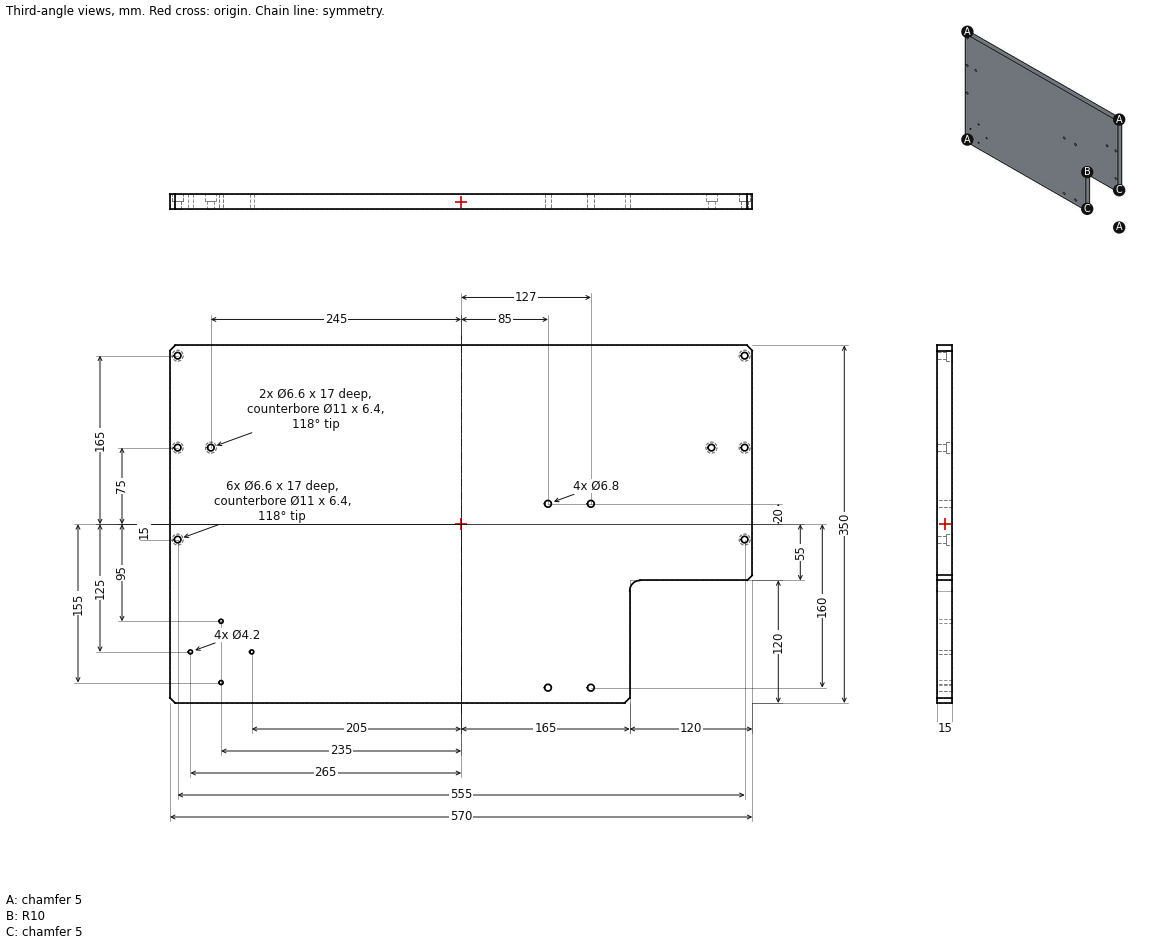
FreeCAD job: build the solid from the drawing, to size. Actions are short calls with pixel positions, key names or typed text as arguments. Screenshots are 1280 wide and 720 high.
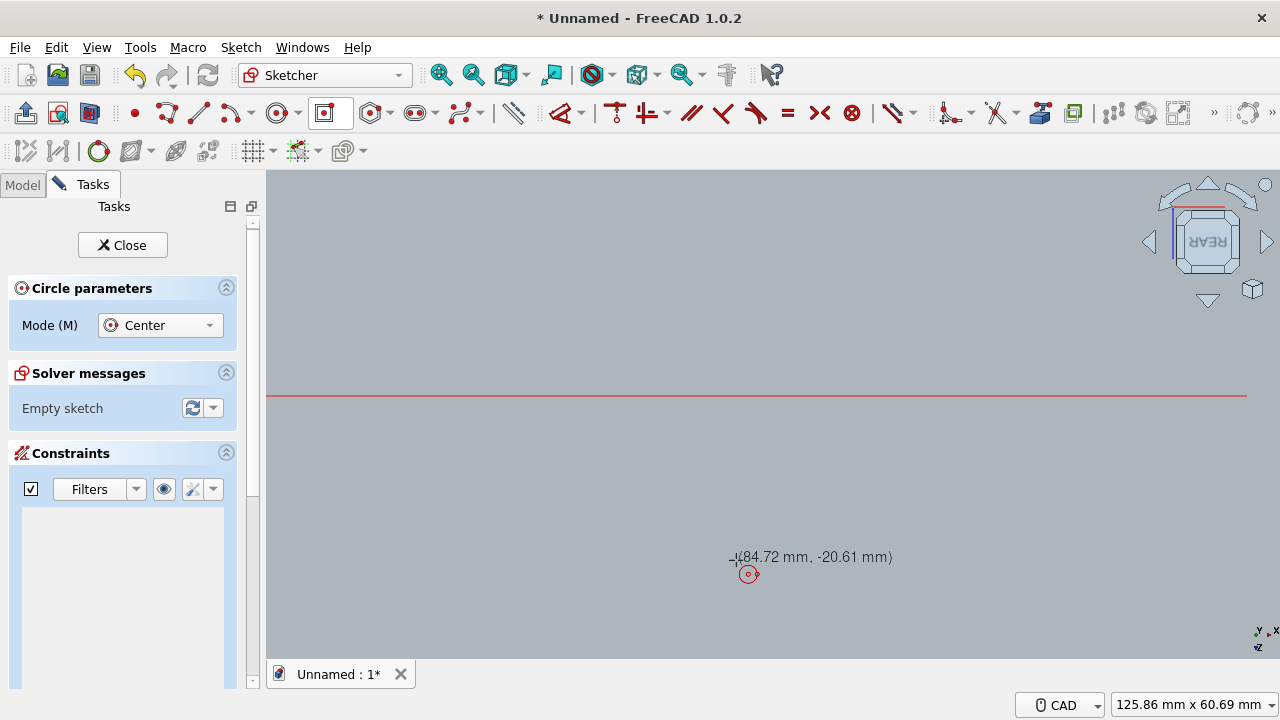
scroll(737, 562, down, 8)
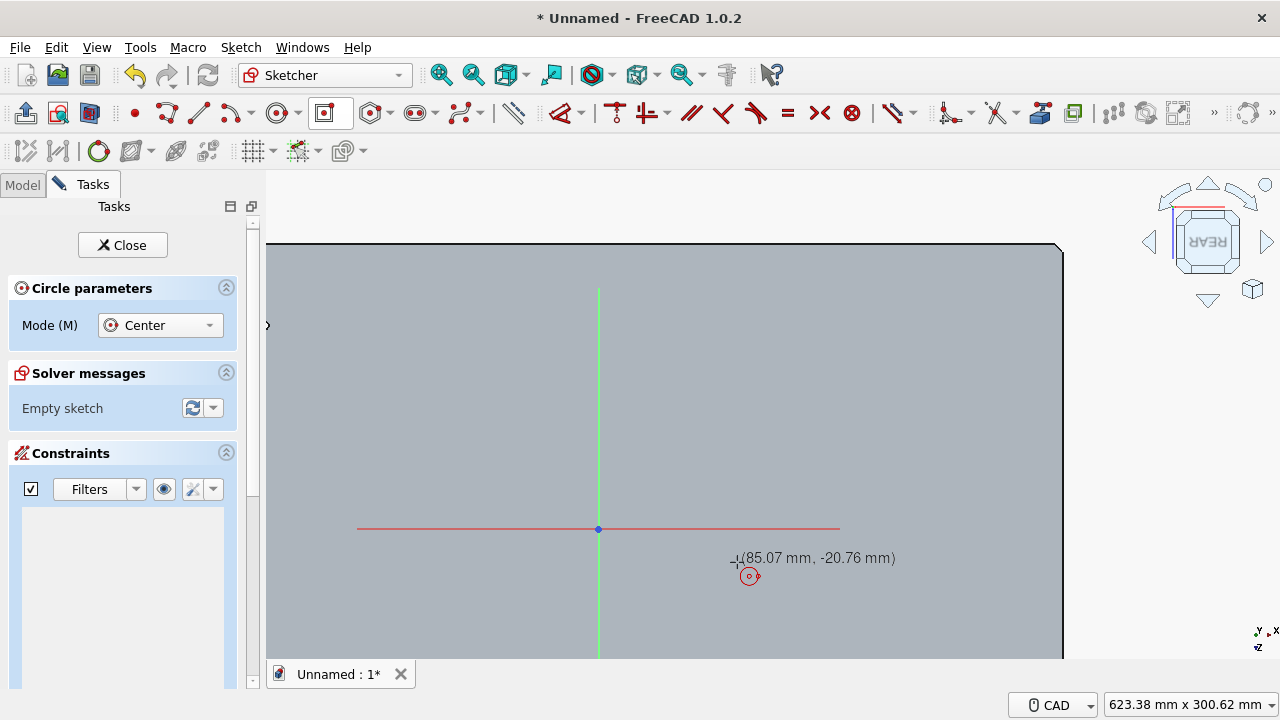
click(737, 562)
move(741, 558)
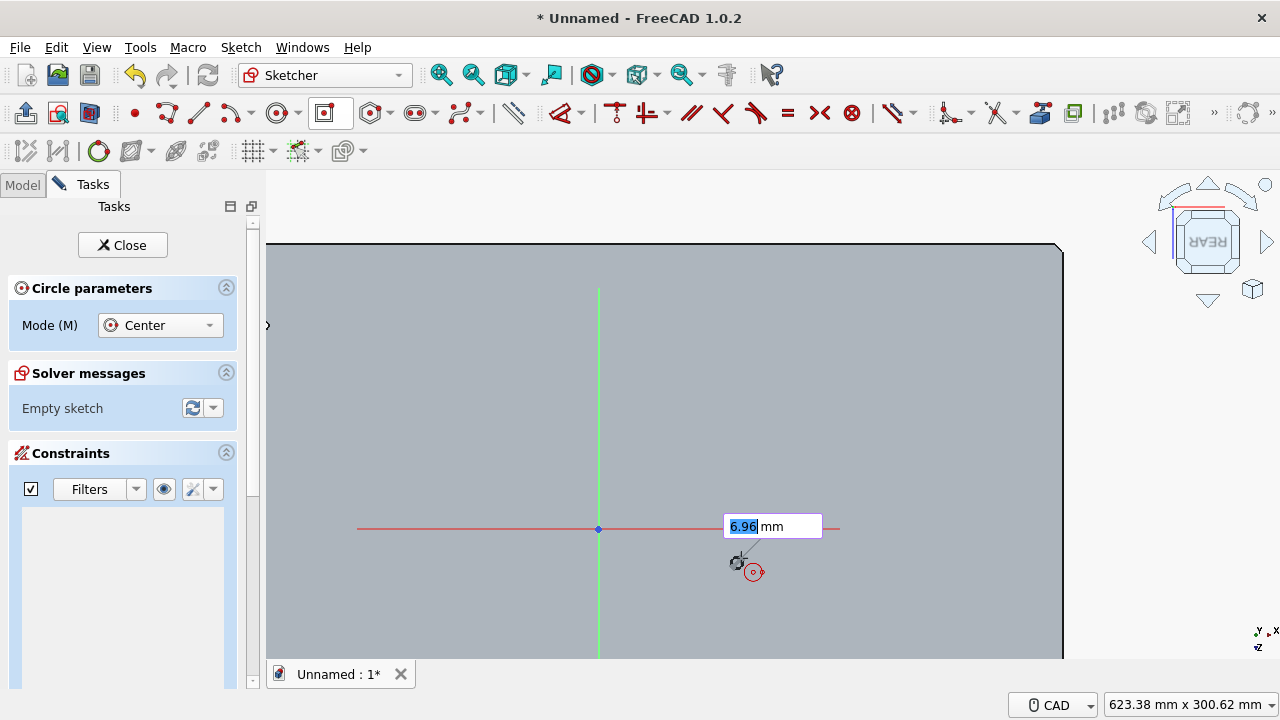
text(6.8)
key(Return)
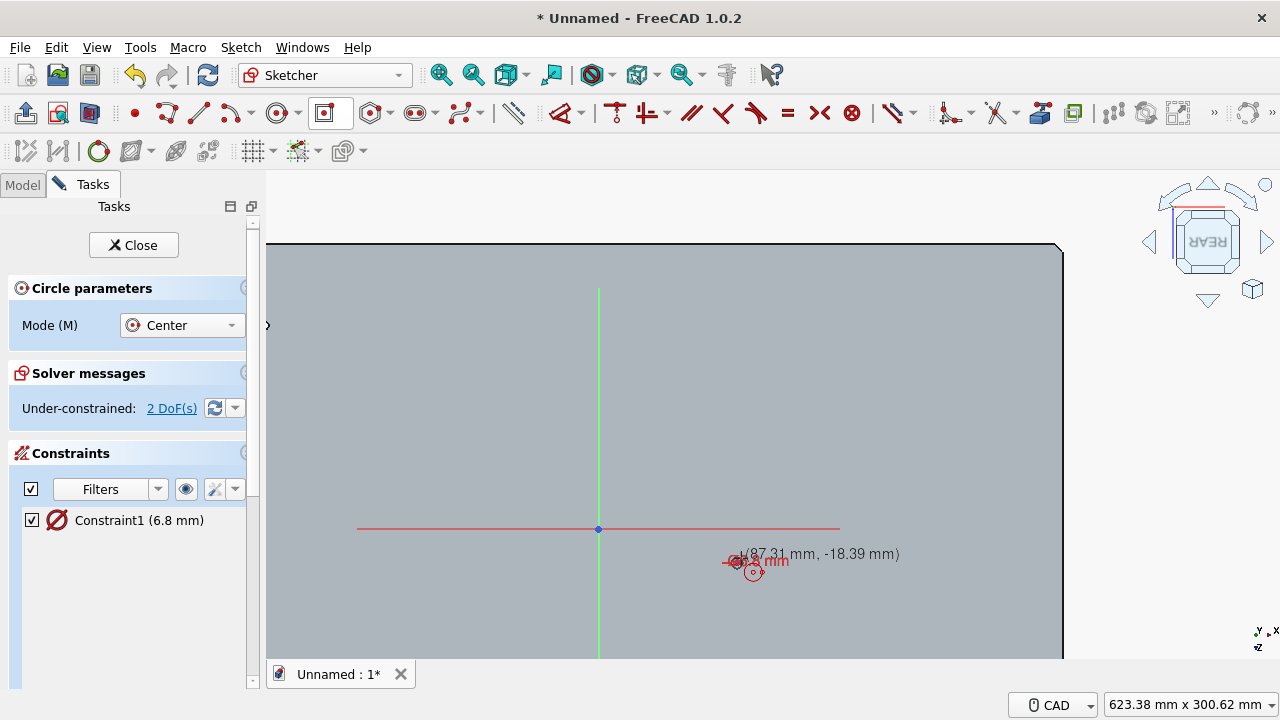
scroll(806, 562, up, 8)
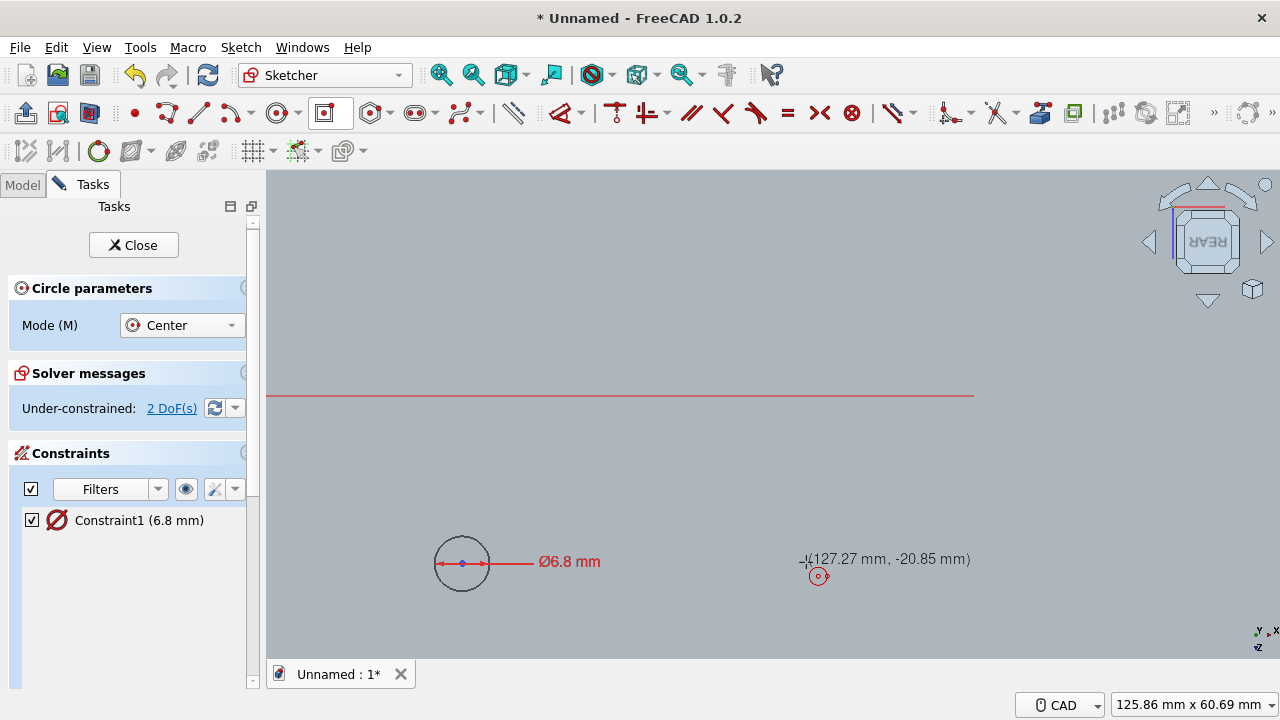
scroll(806, 562, down, 8)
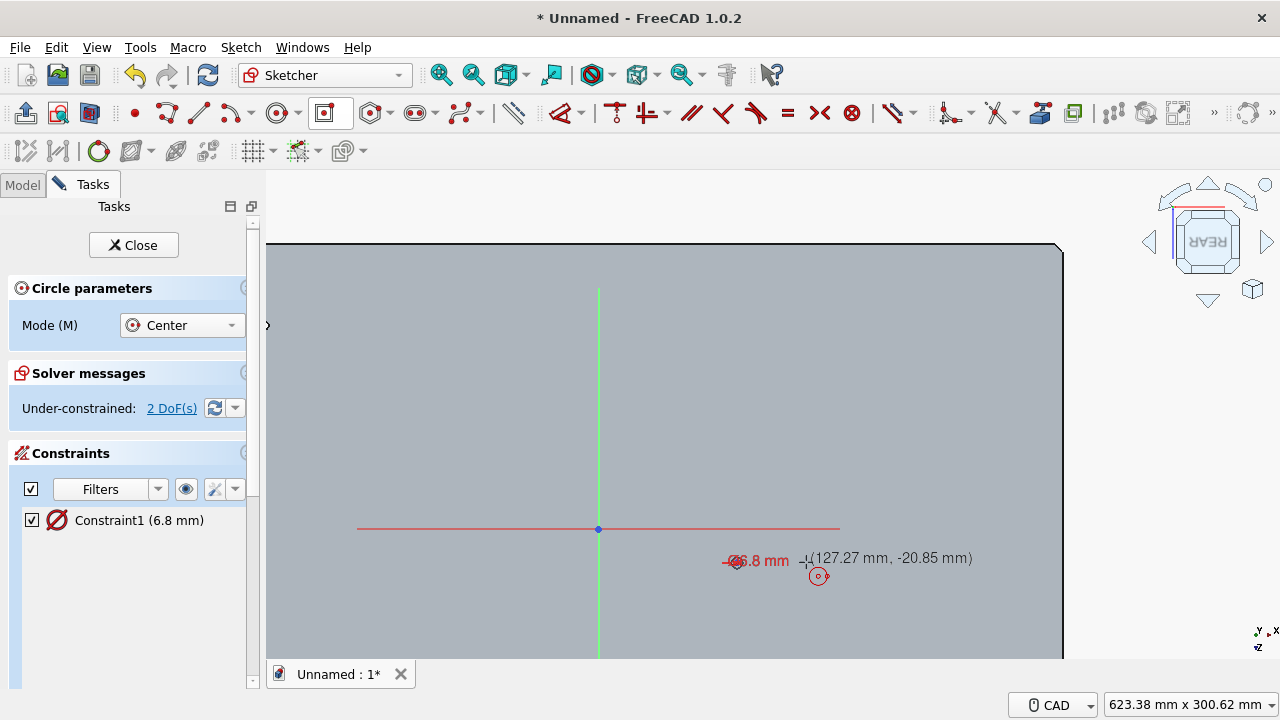
click(806, 562)
move(809, 558)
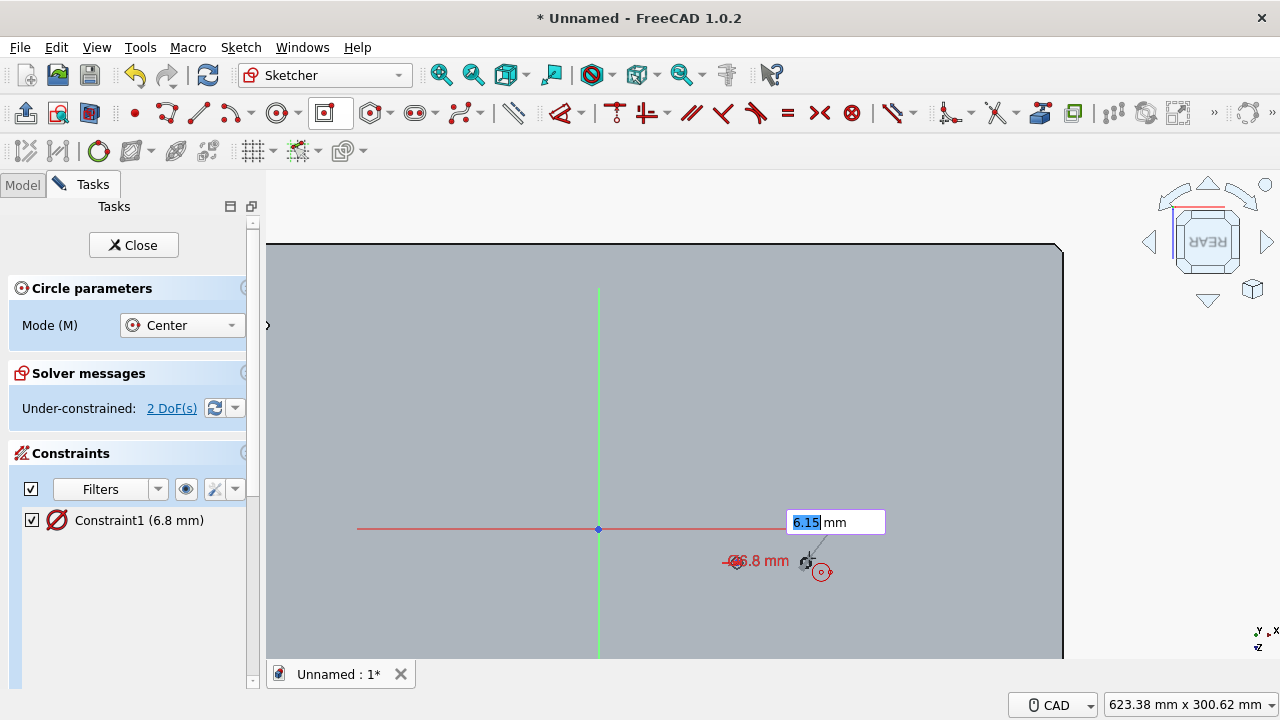
text(6.8)
key(Return)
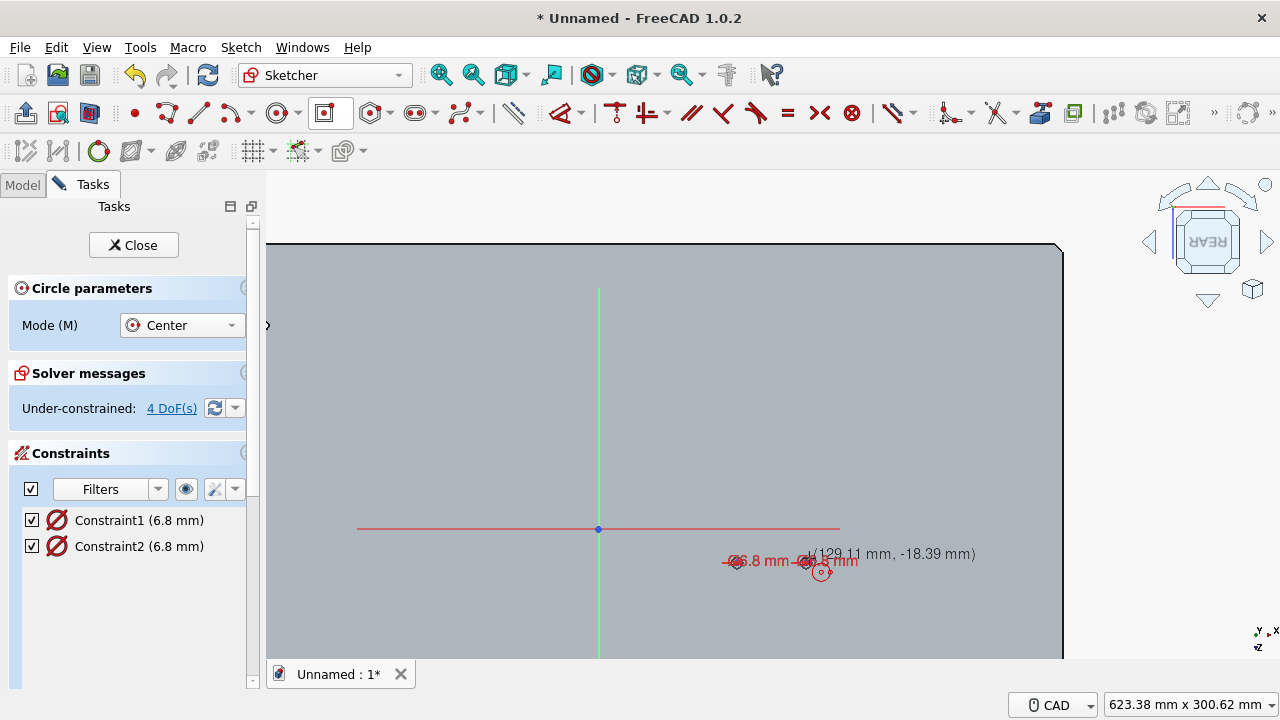
scroll(806, 269, up, 8)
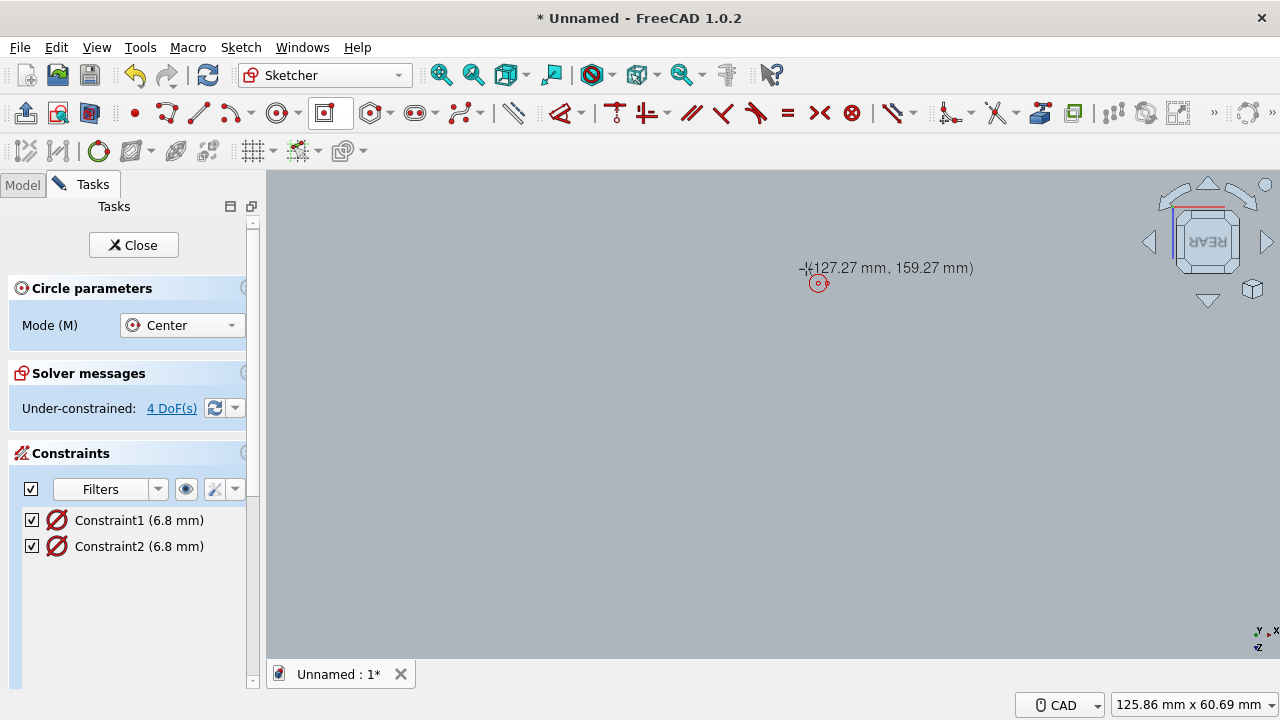
scroll(806, 268, down, 8)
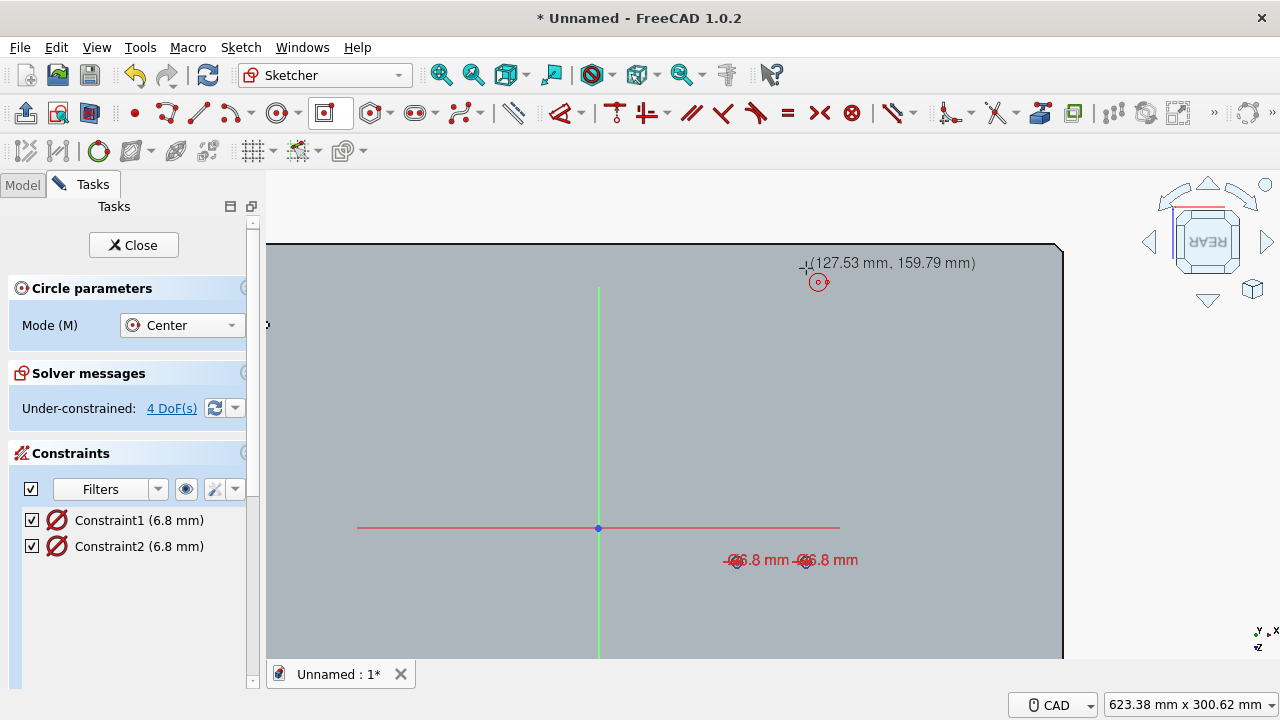
click(806, 268)
move(809, 264)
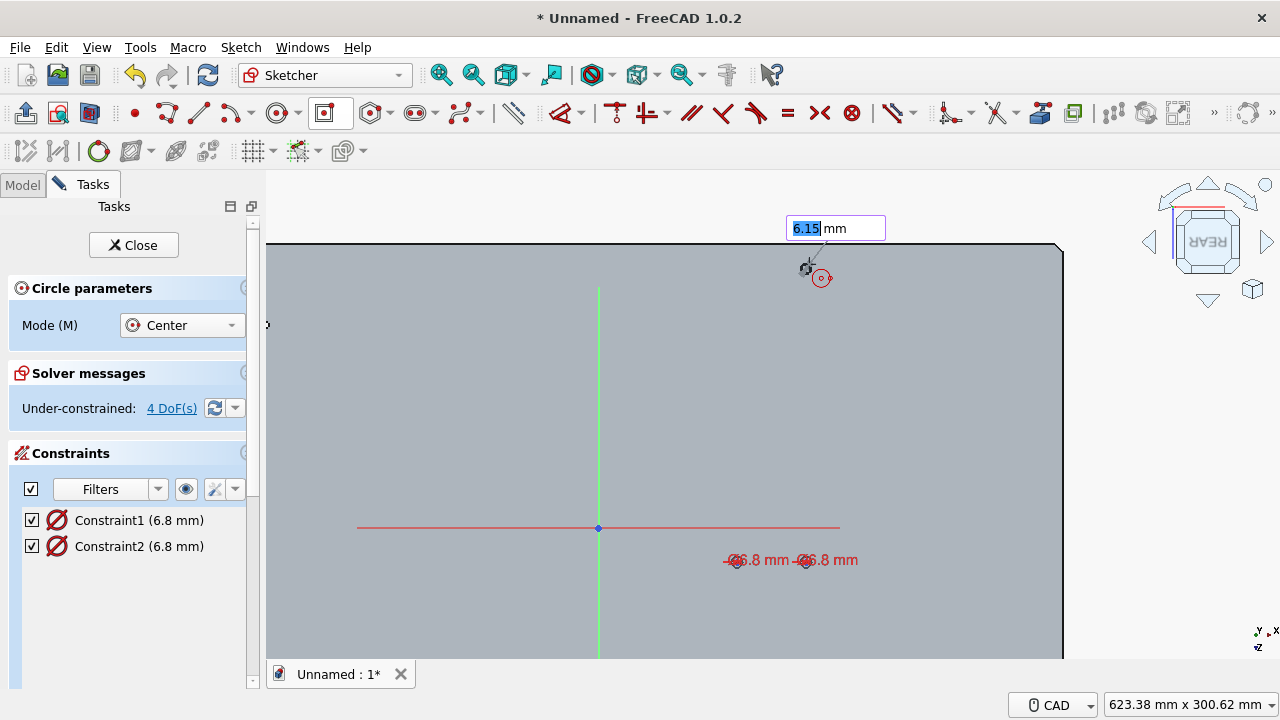
text(6.8)
key(Return)